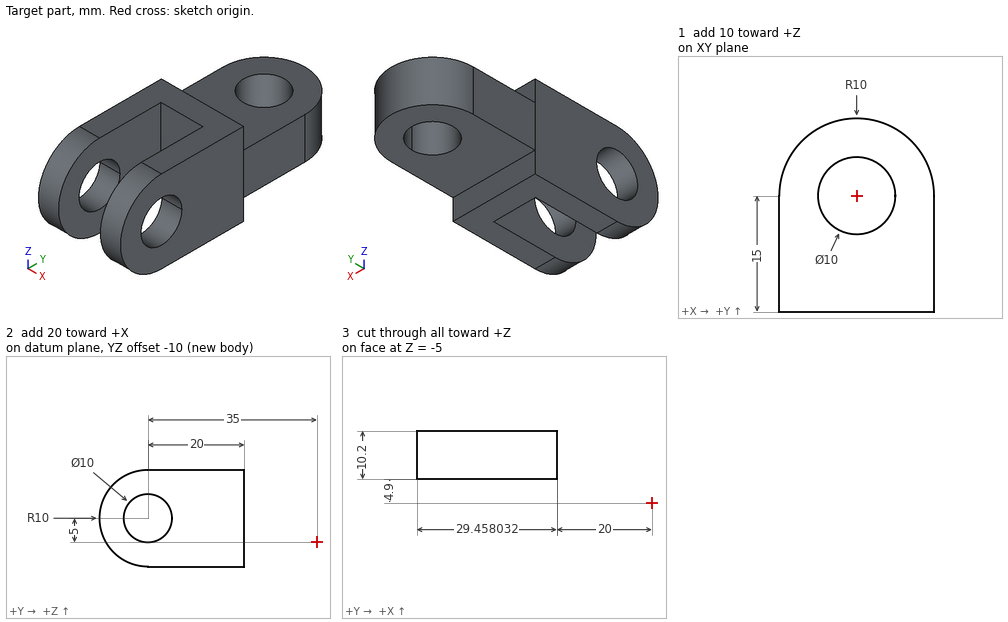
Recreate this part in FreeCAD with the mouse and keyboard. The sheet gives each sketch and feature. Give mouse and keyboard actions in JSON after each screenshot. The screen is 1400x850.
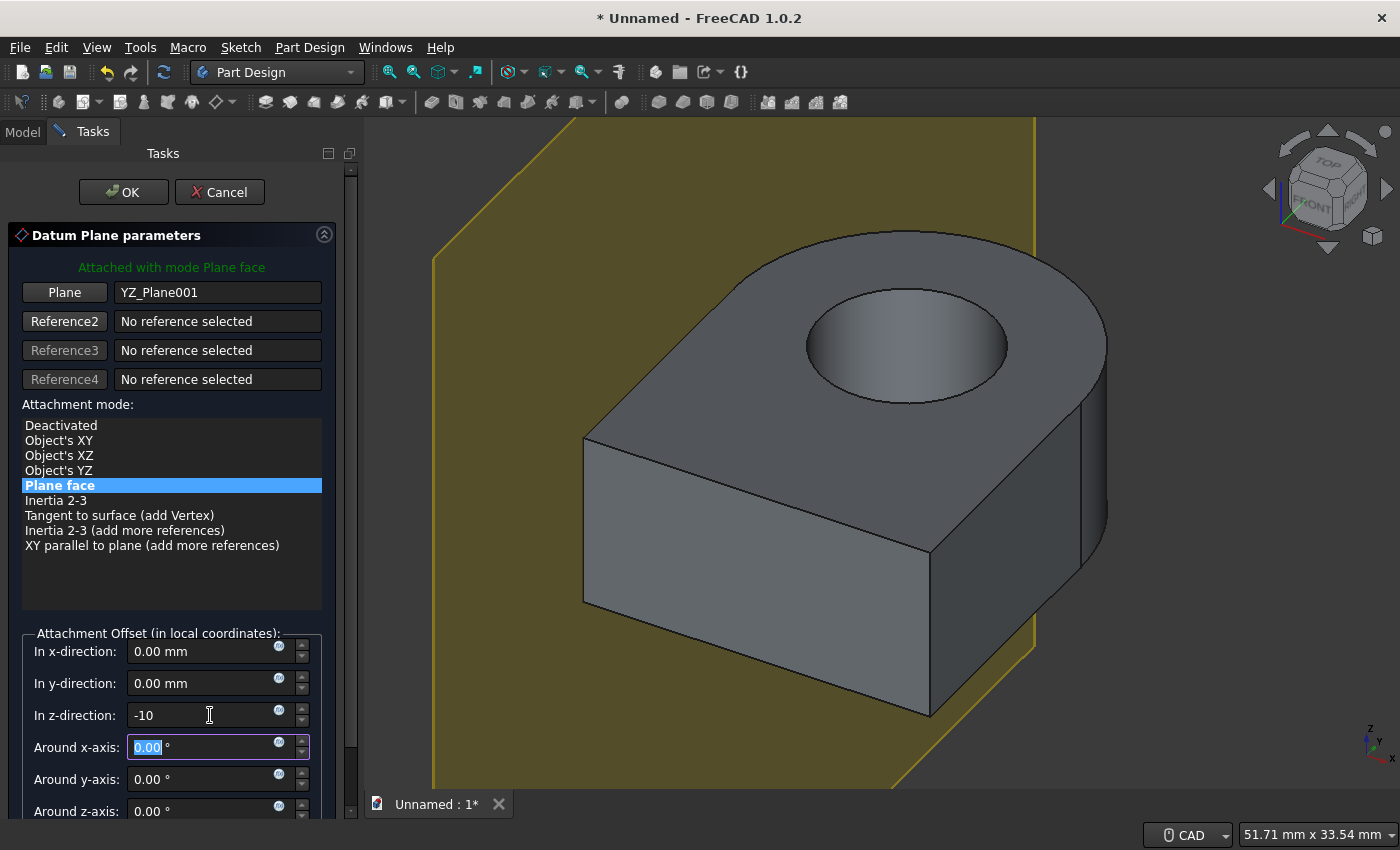
{"action": "left_click", "coordinate": [124, 192]}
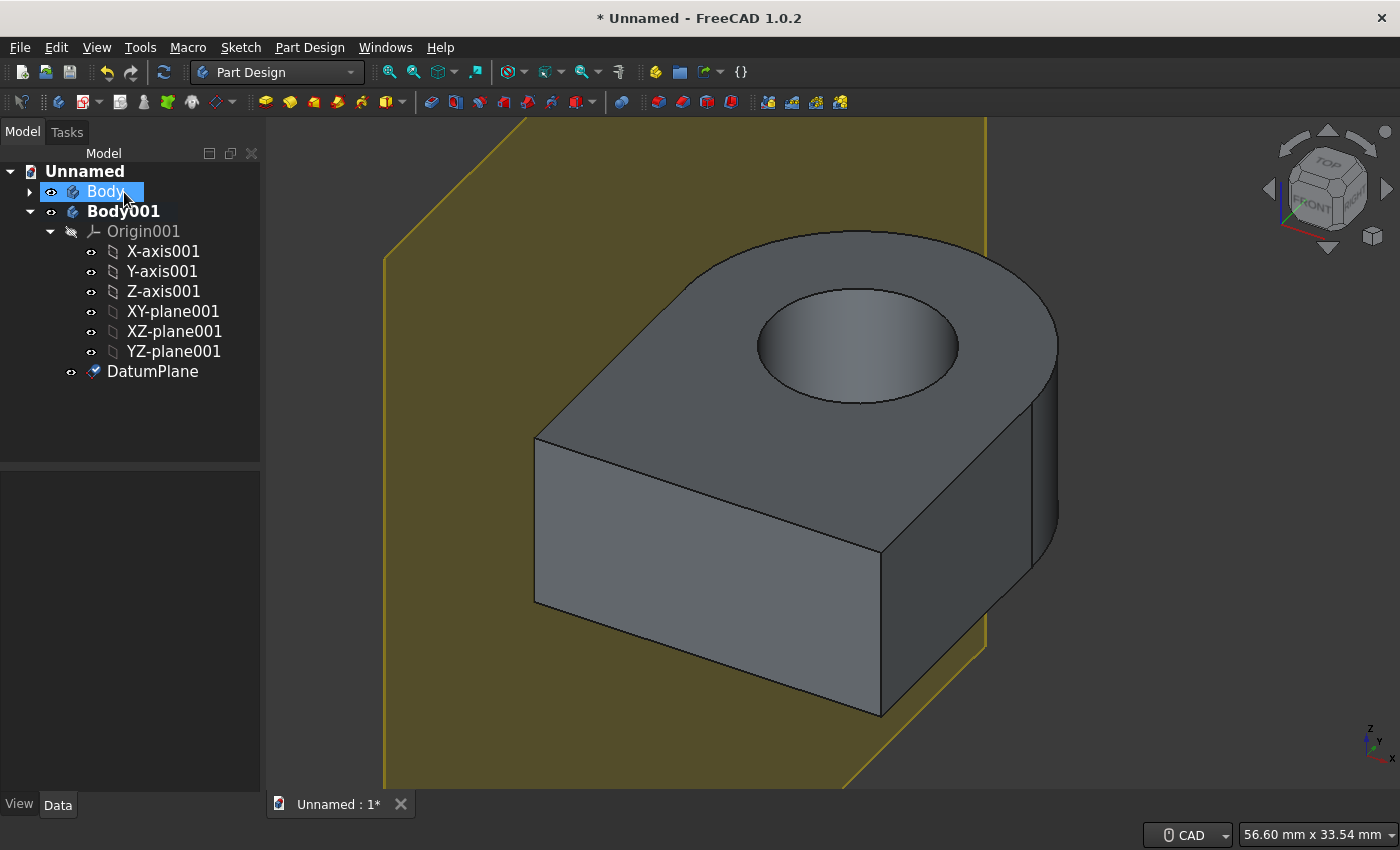
{"action": "left_click", "coordinate": [116, 372]}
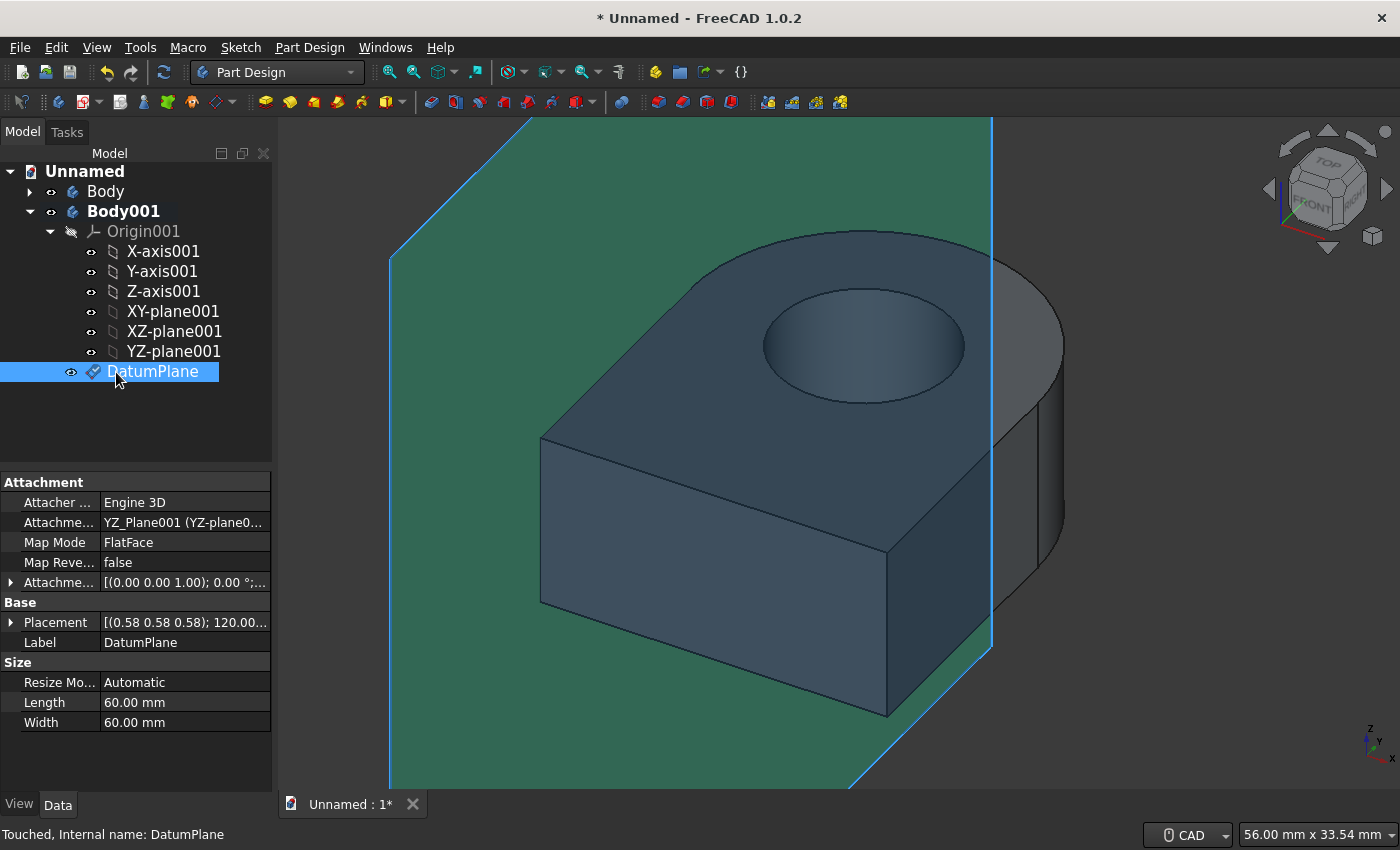
{"action": "left_click", "coordinate": [84, 102]}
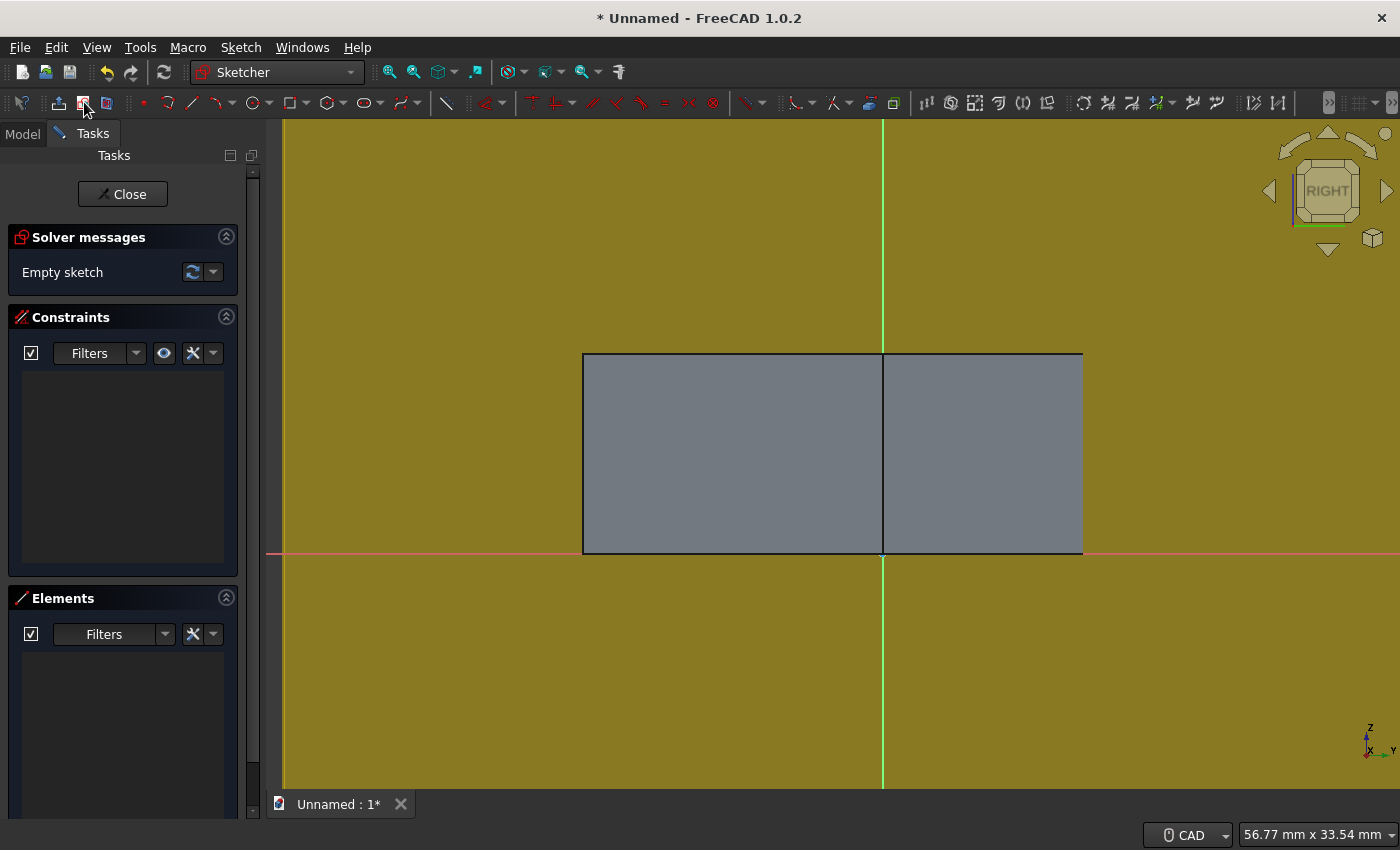
{"action": "scroll", "coordinate": [1235, 454], "scroll_direction": "down", "scroll_amount": 2}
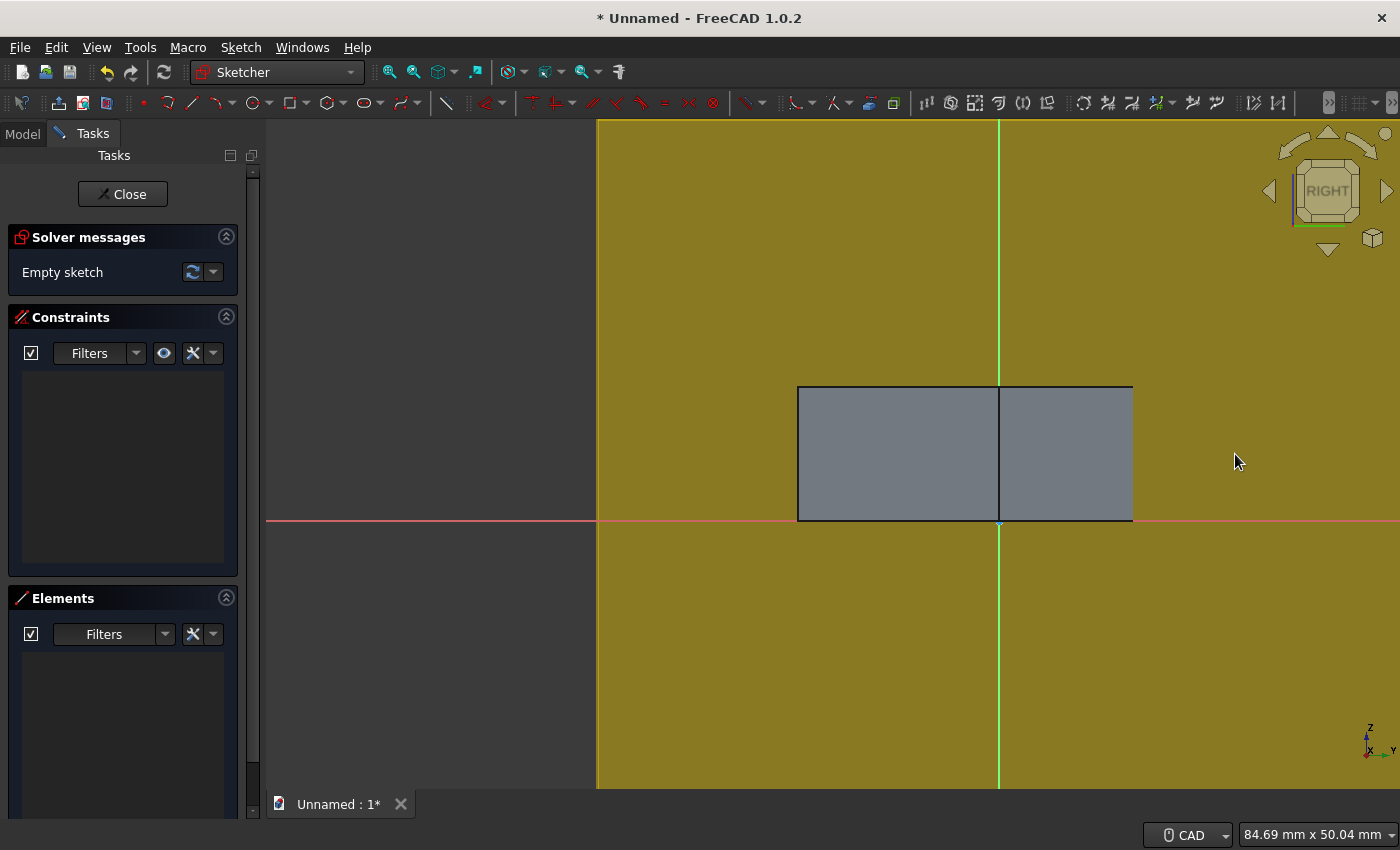
{"action": "left_click", "coordinate": [168, 104]}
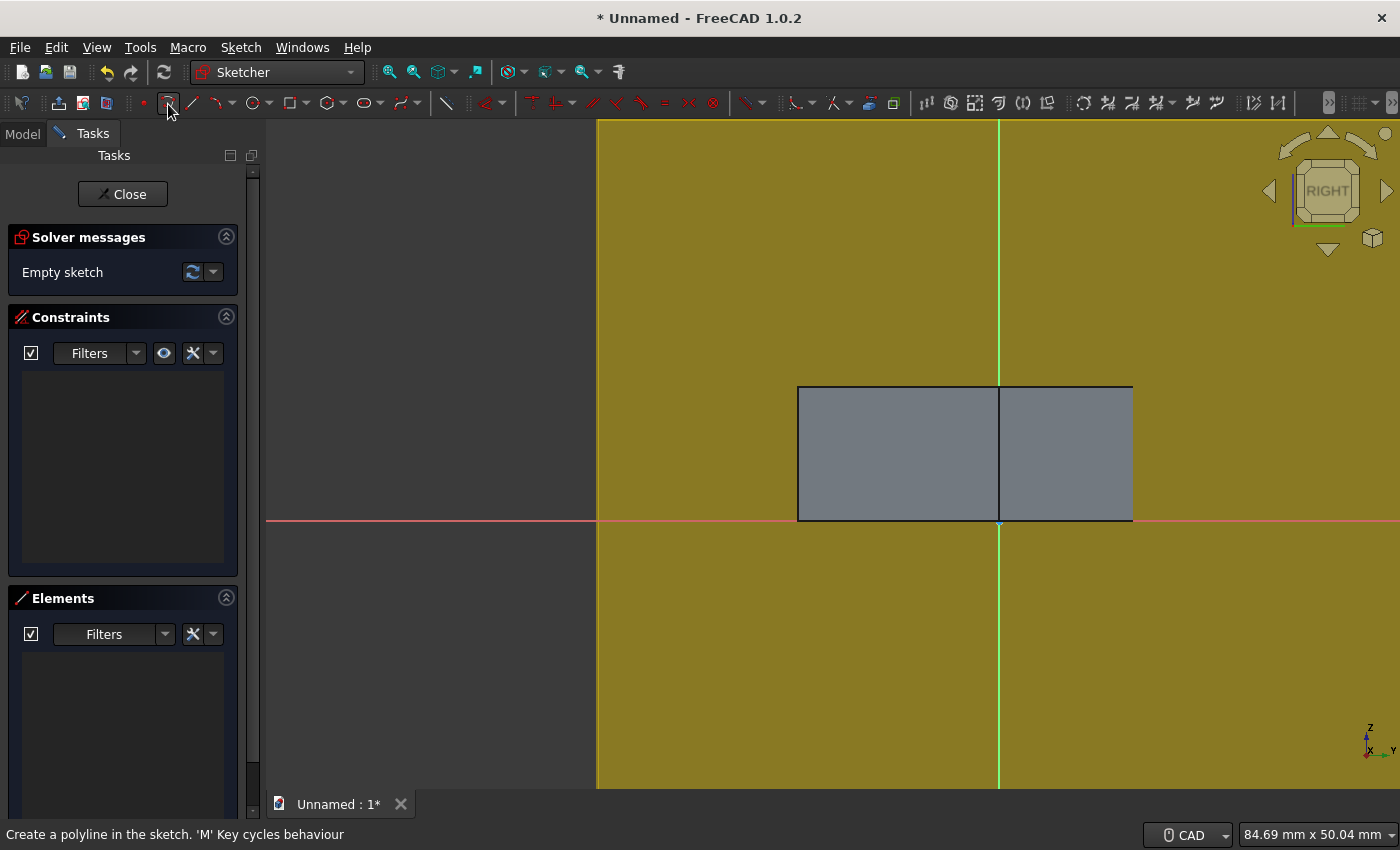
{"action": "left_click", "coordinate": [531, 320]}
{"action": "left_click", "coordinate": [798, 320]}
{"action": "left_click", "coordinate": [798, 588]}
{"action": "left_click", "coordinate": [531, 588]}
{"action": "right_click", "coordinate": [531, 588]}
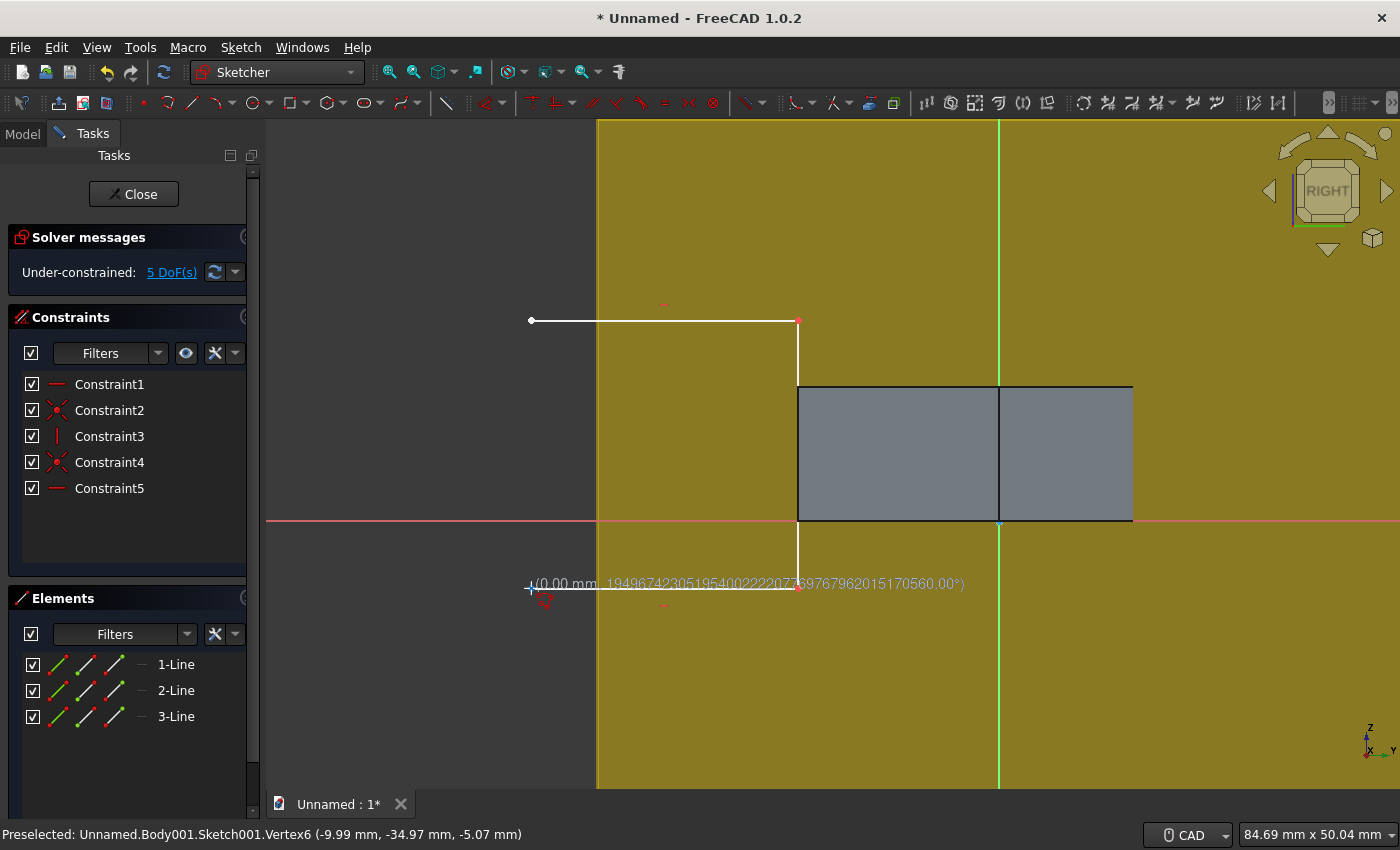
{"action": "left_click", "coordinate": [216, 104]}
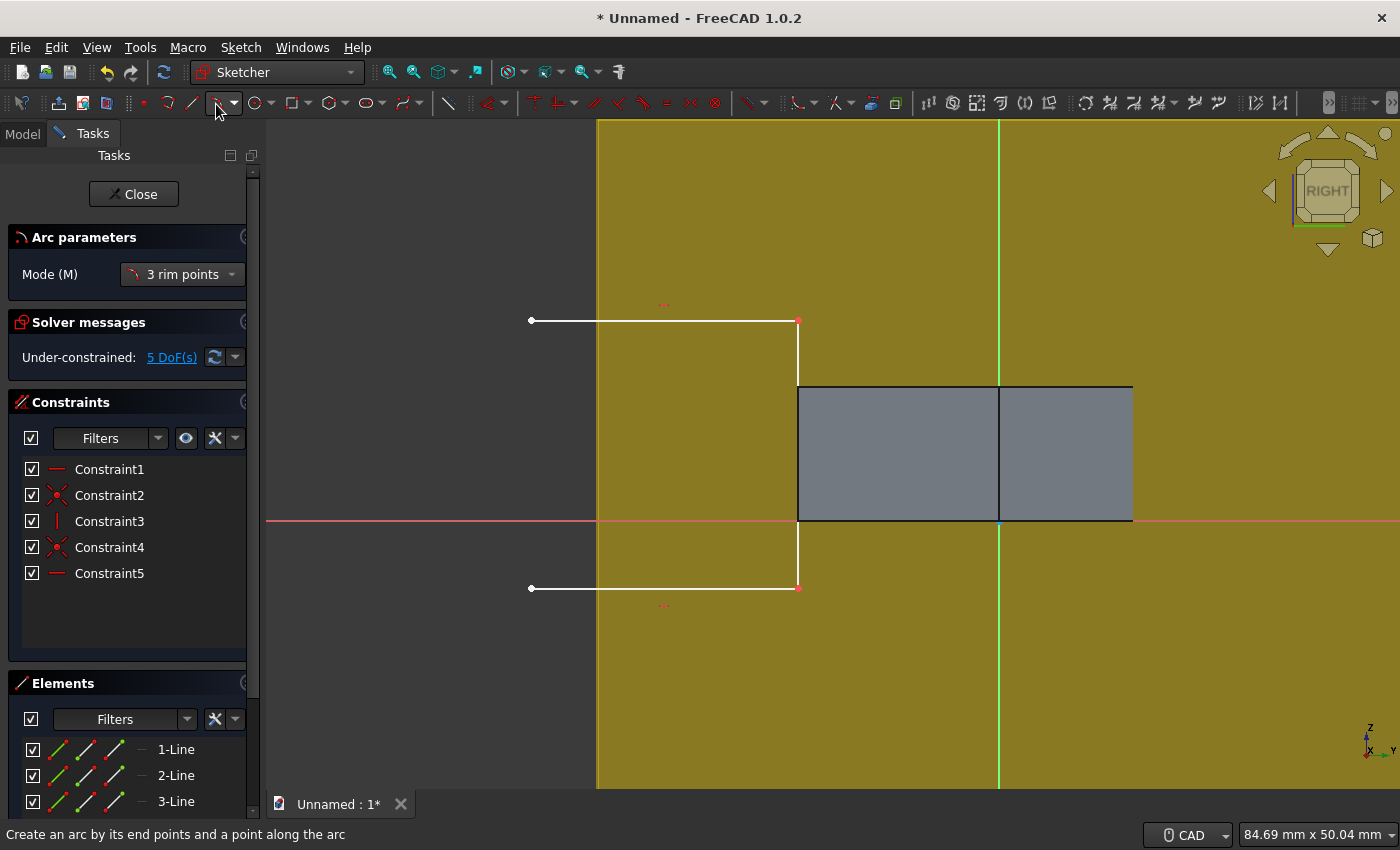
{"action": "left_click", "coordinate": [531, 589]}
{"action": "left_click", "coordinate": [531, 321]}
{"action": "left_click", "coordinate": [397, 454]}